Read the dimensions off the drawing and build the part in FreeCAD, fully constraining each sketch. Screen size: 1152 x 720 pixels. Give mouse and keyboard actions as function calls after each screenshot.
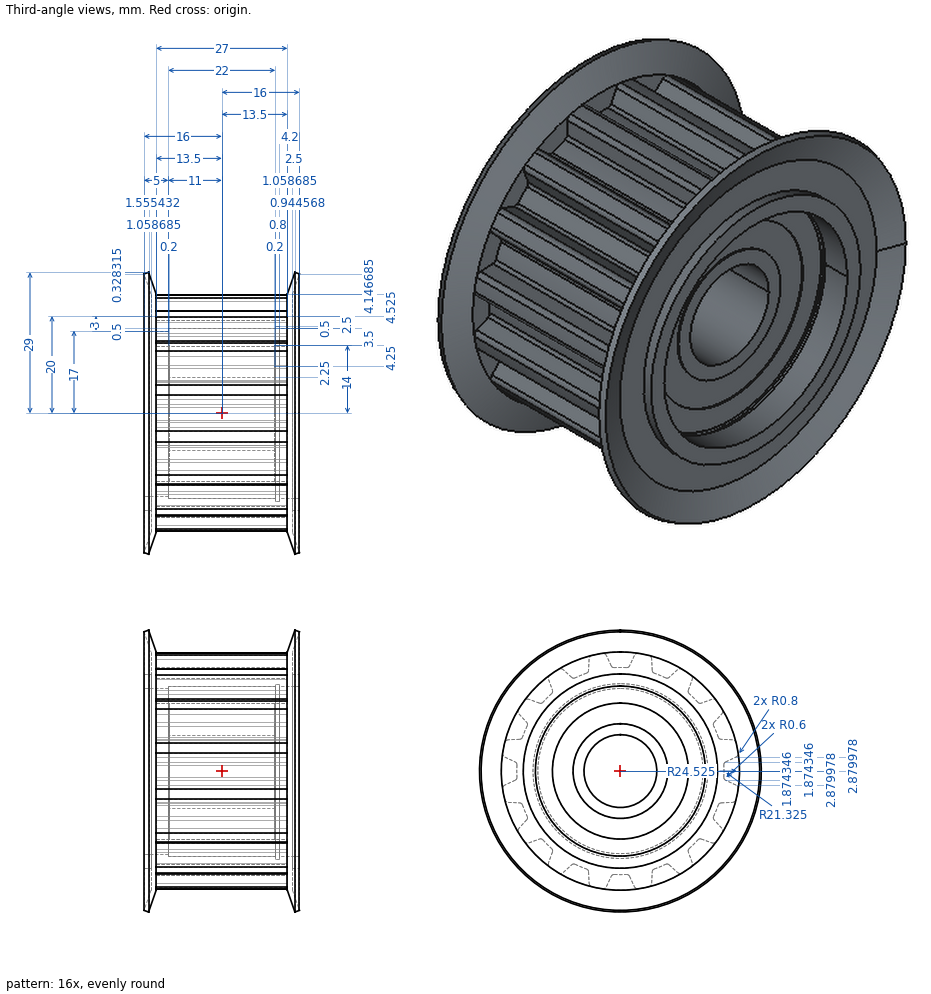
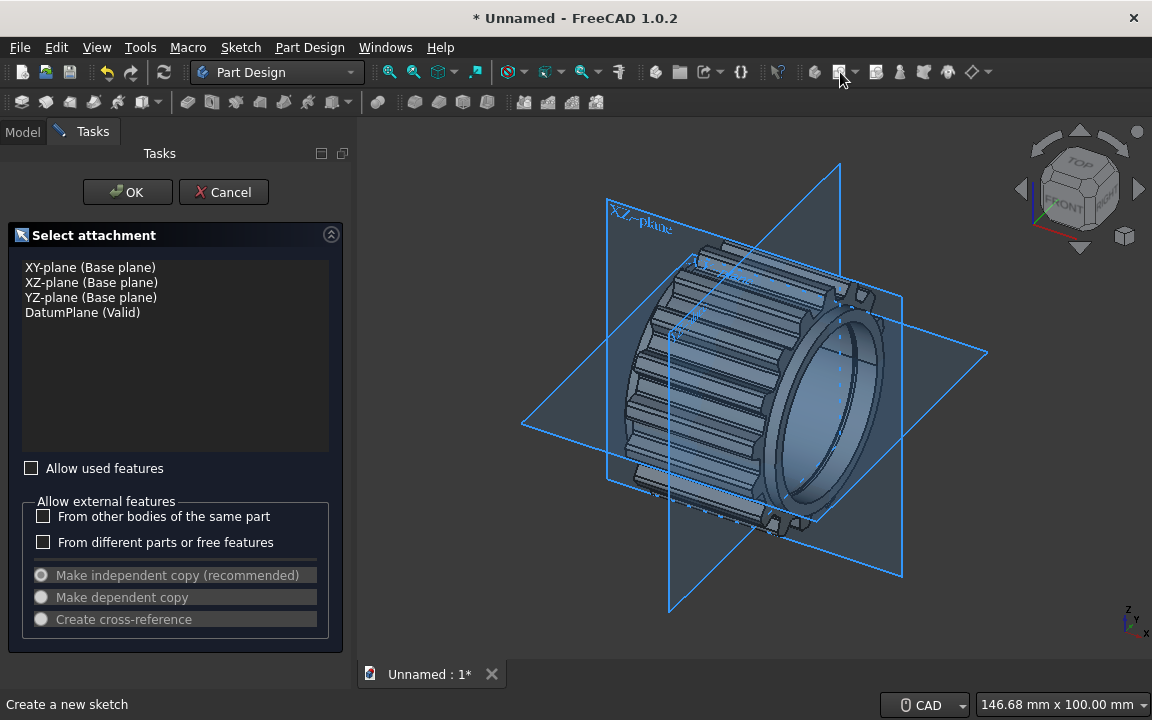
click(82, 268)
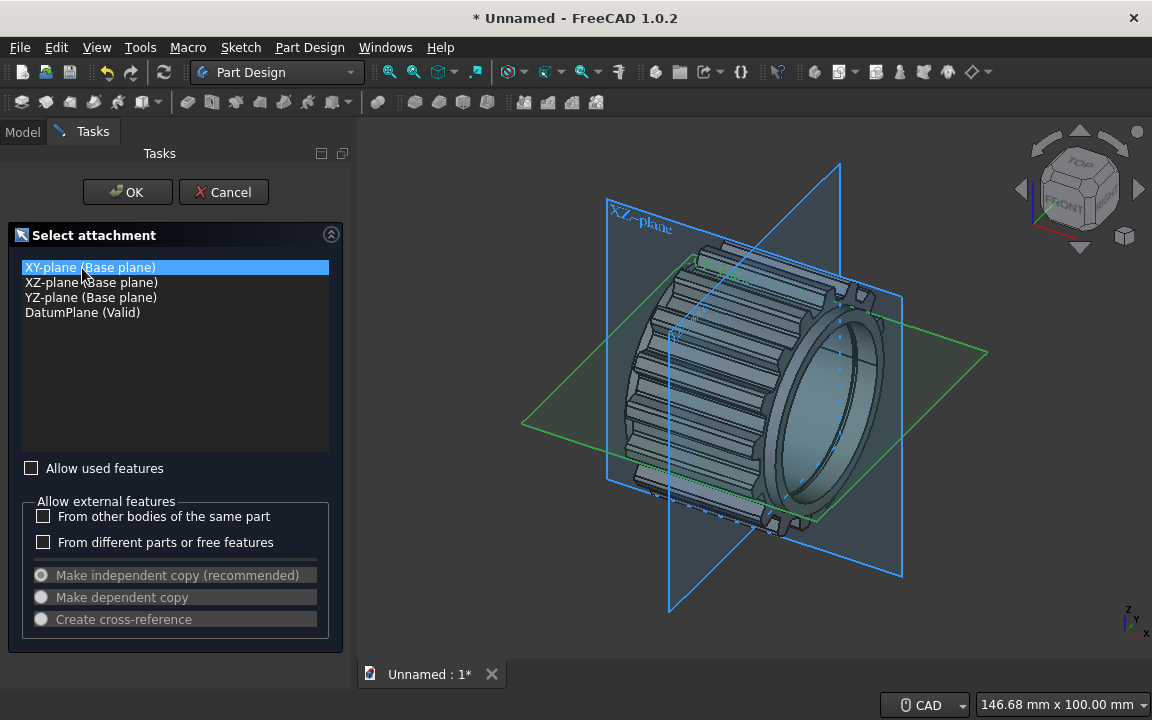
click(128, 192)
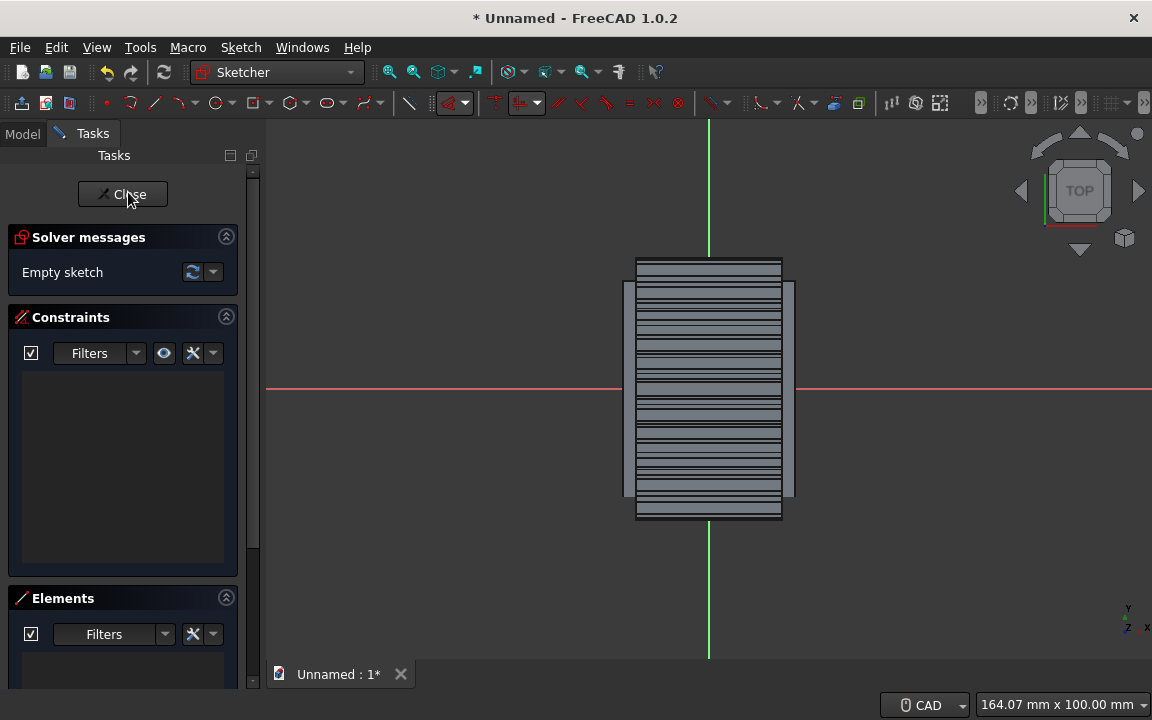
click(70, 104)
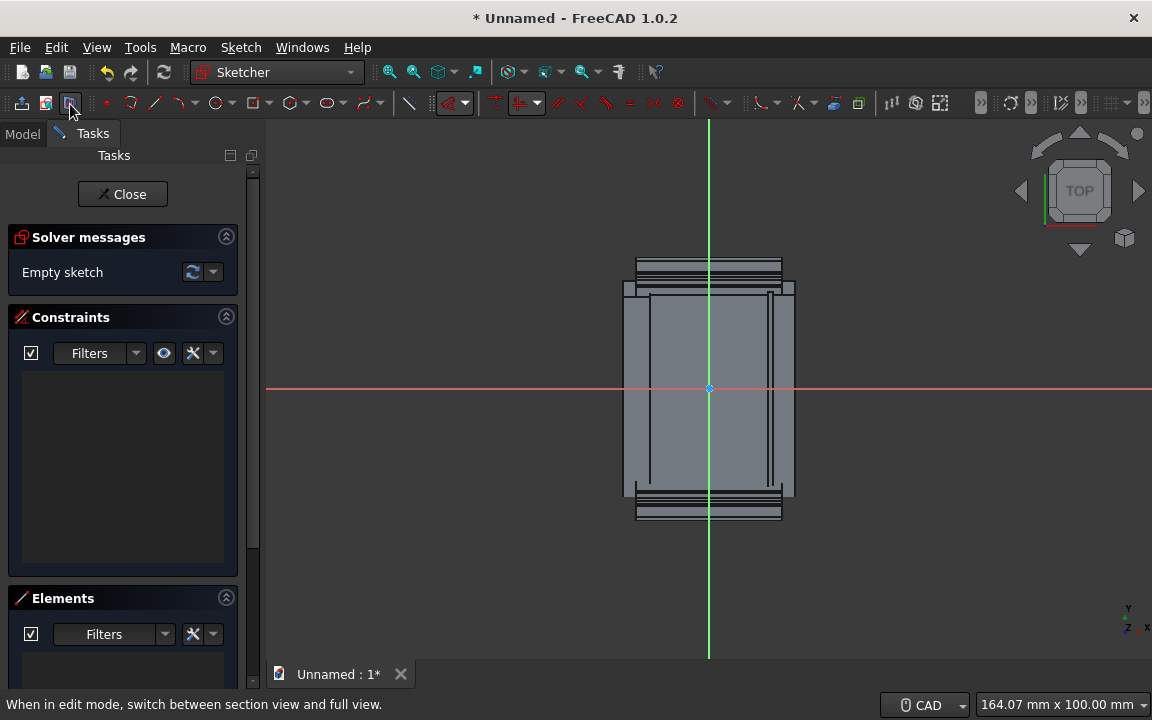
scroll(628, 236, up, 10)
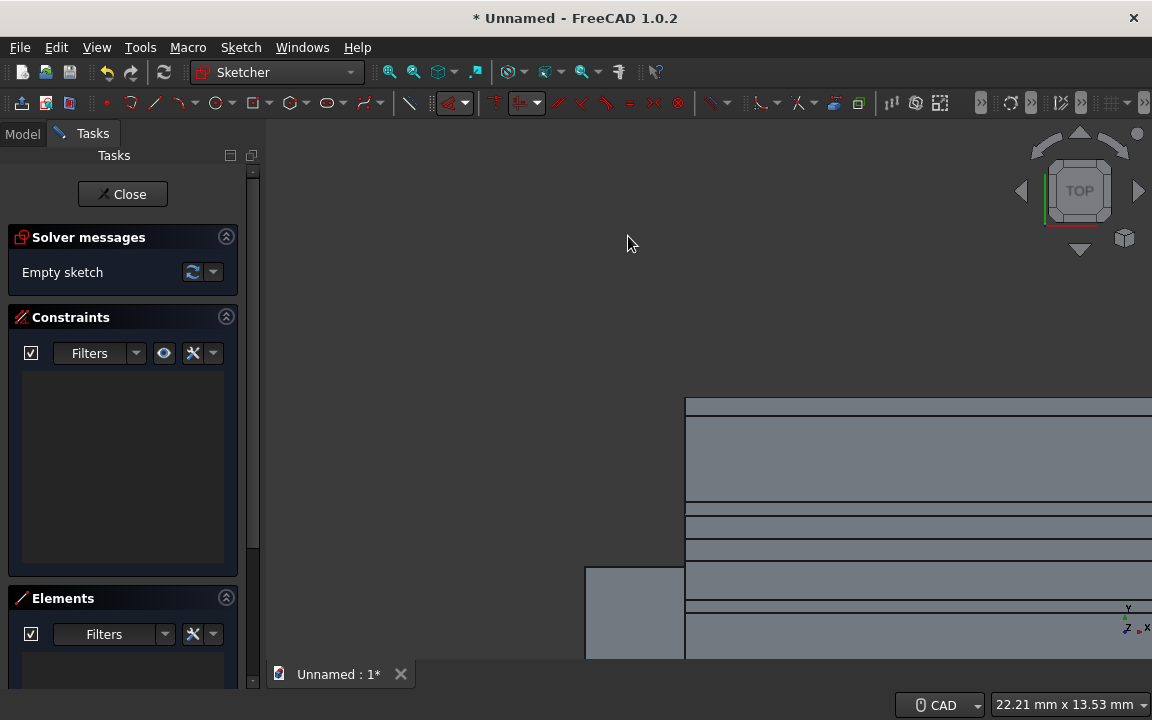
click(132, 104)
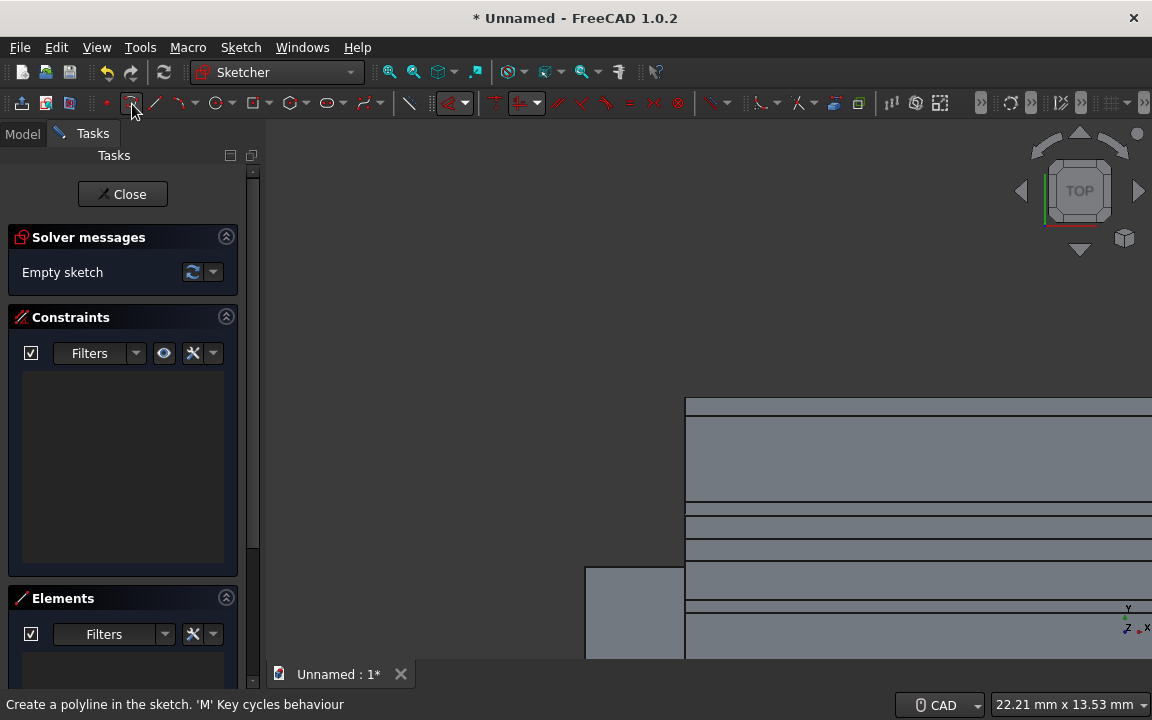
click(685, 567)
click(685, 387)
click(623, 208)
click(585, 221)
click(643, 387)
click(643, 567)
click(685, 568)
key(Escape)
key(Escape)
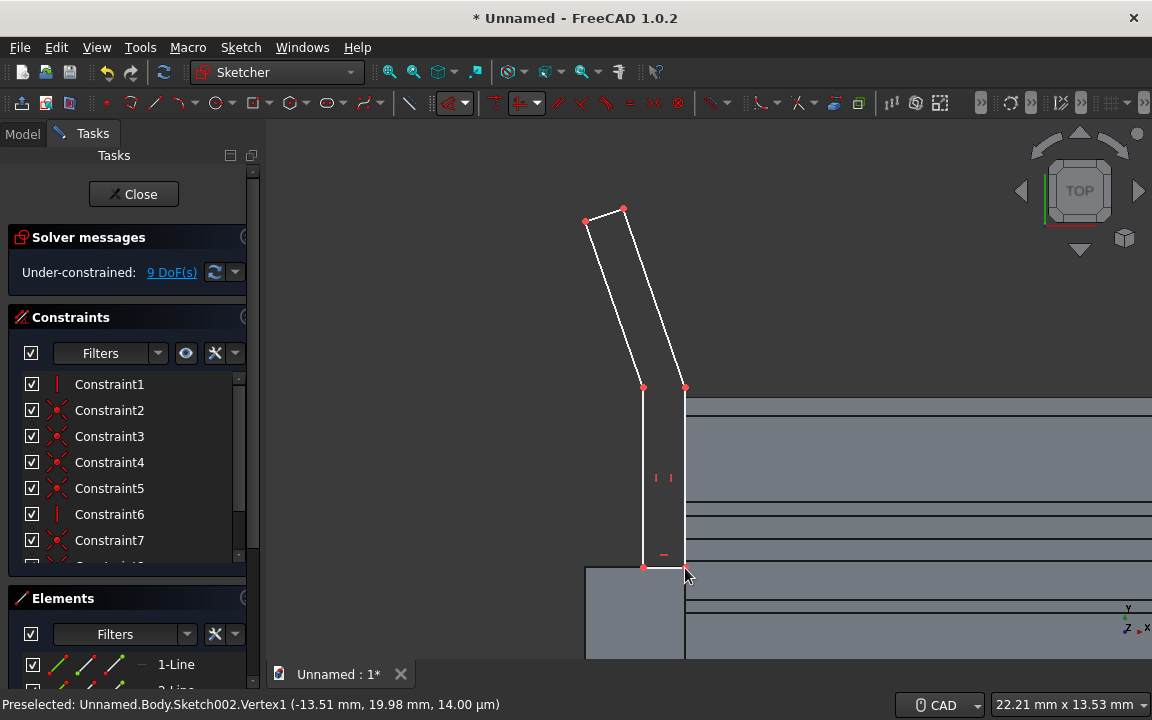
click(685, 568)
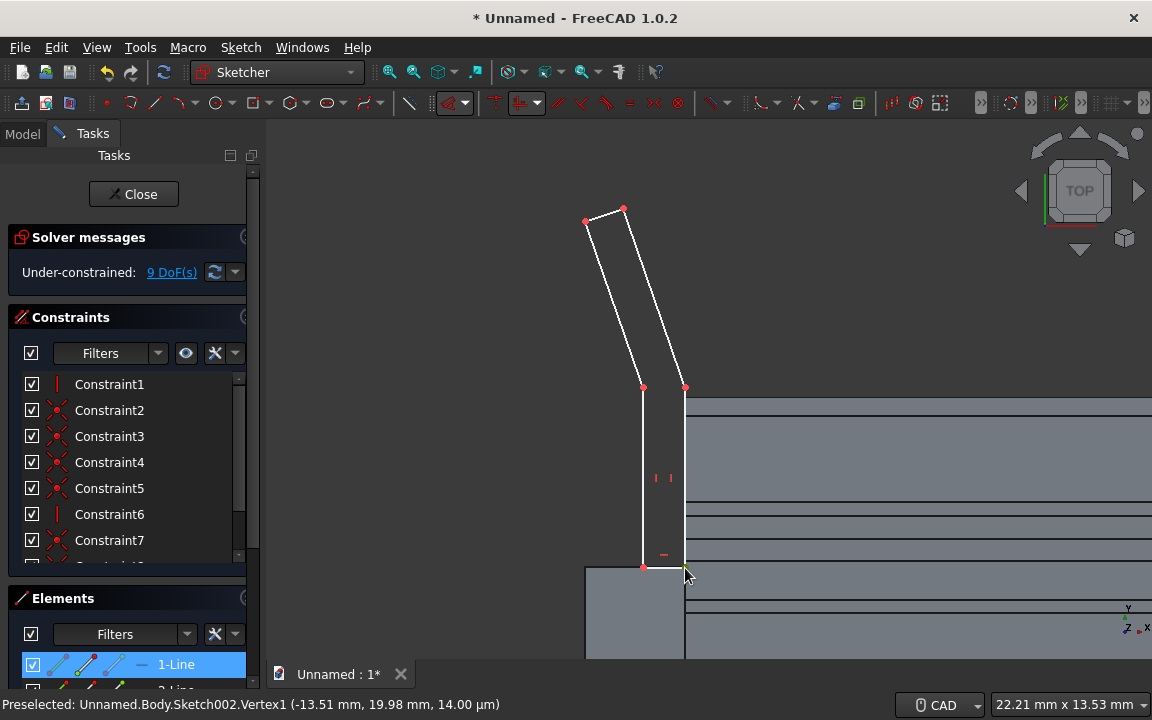
click(468, 104)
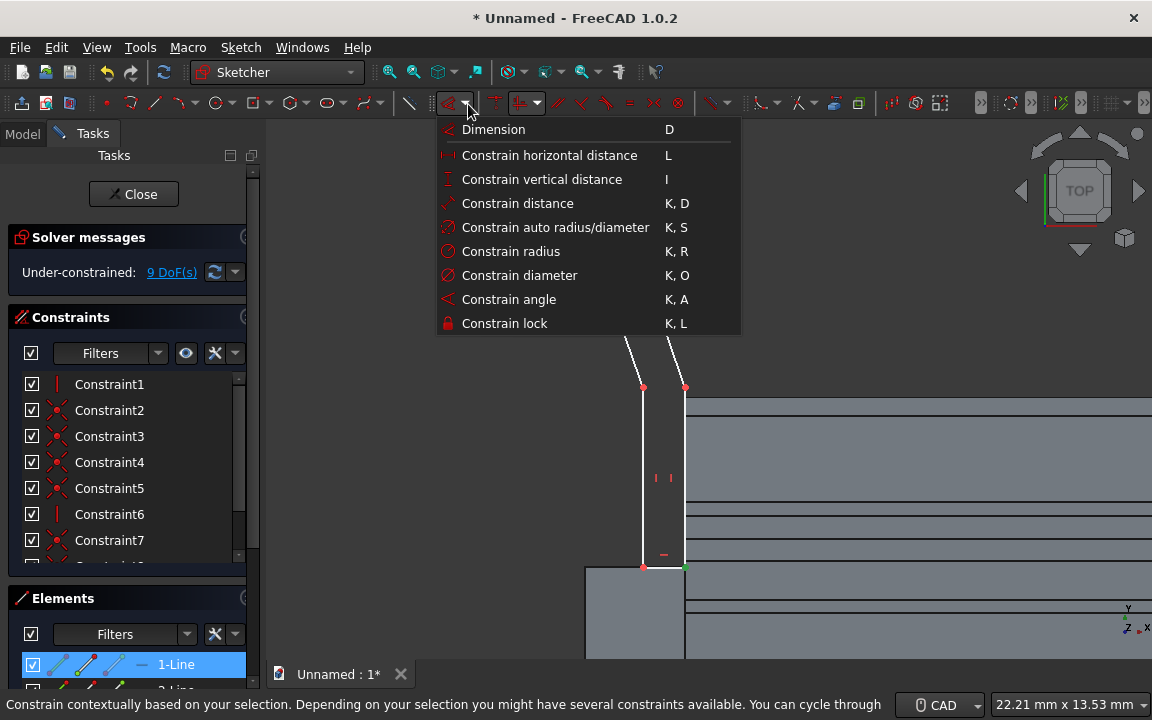
click(589, 179)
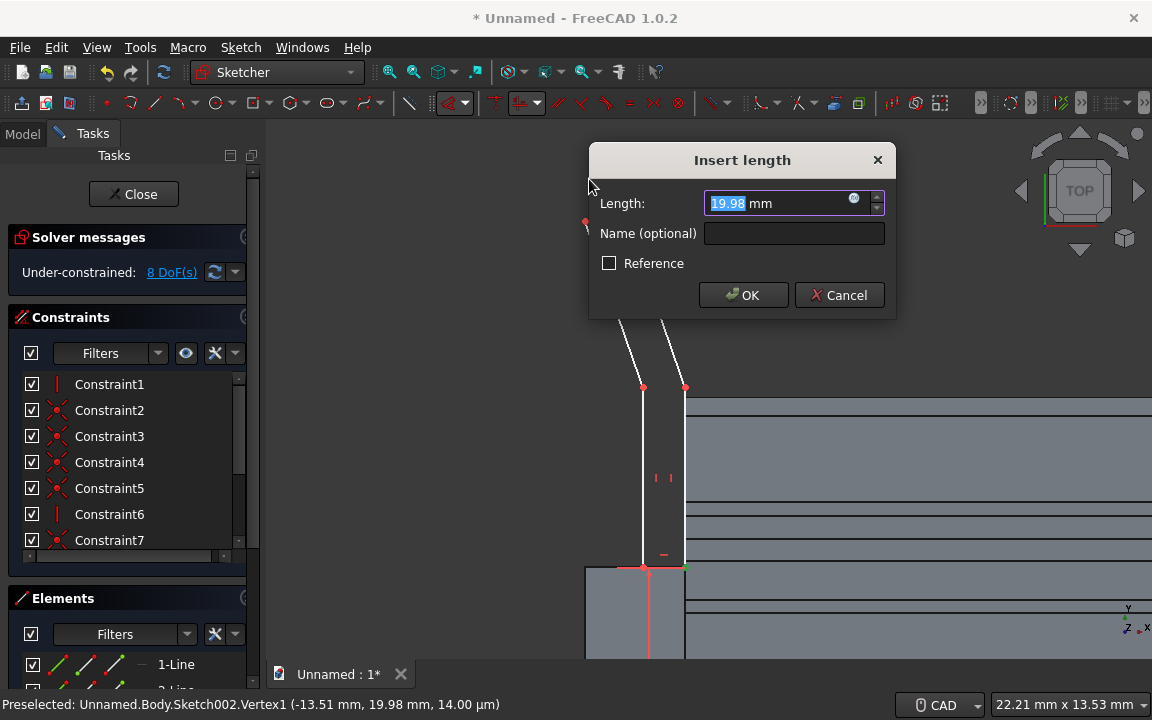
text(20)
key(Return)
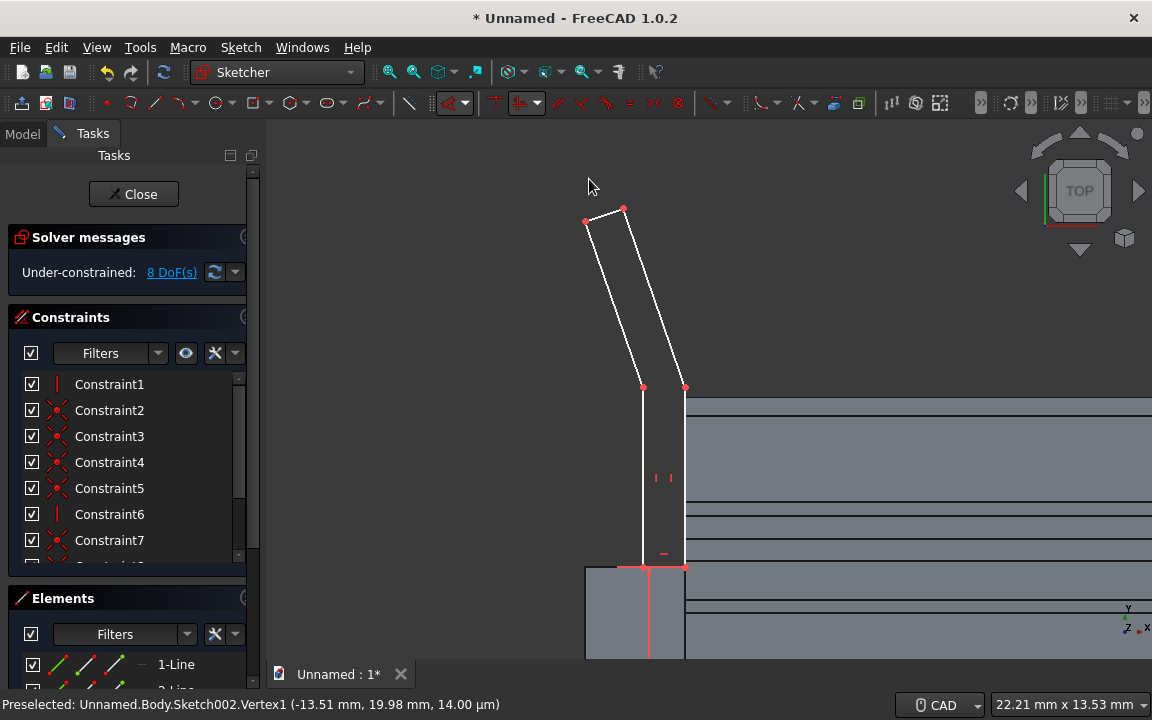
click(623, 209)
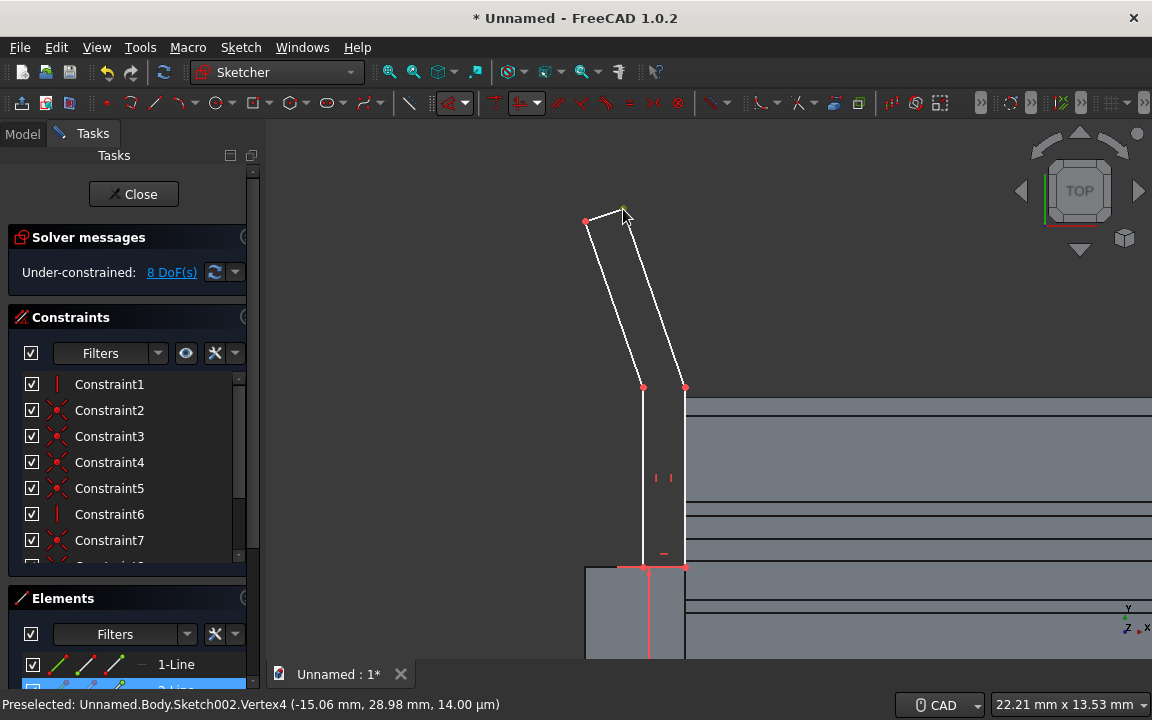
key(i)